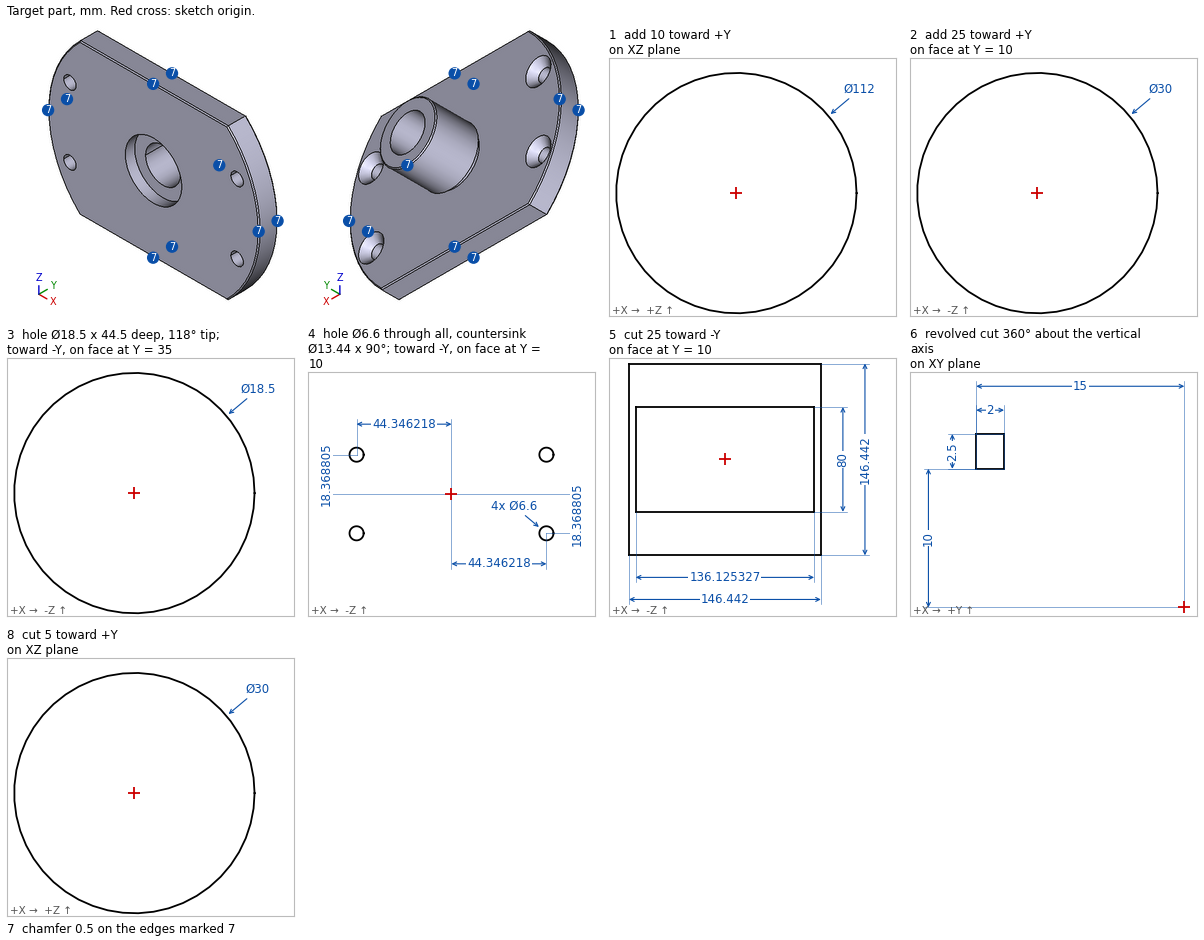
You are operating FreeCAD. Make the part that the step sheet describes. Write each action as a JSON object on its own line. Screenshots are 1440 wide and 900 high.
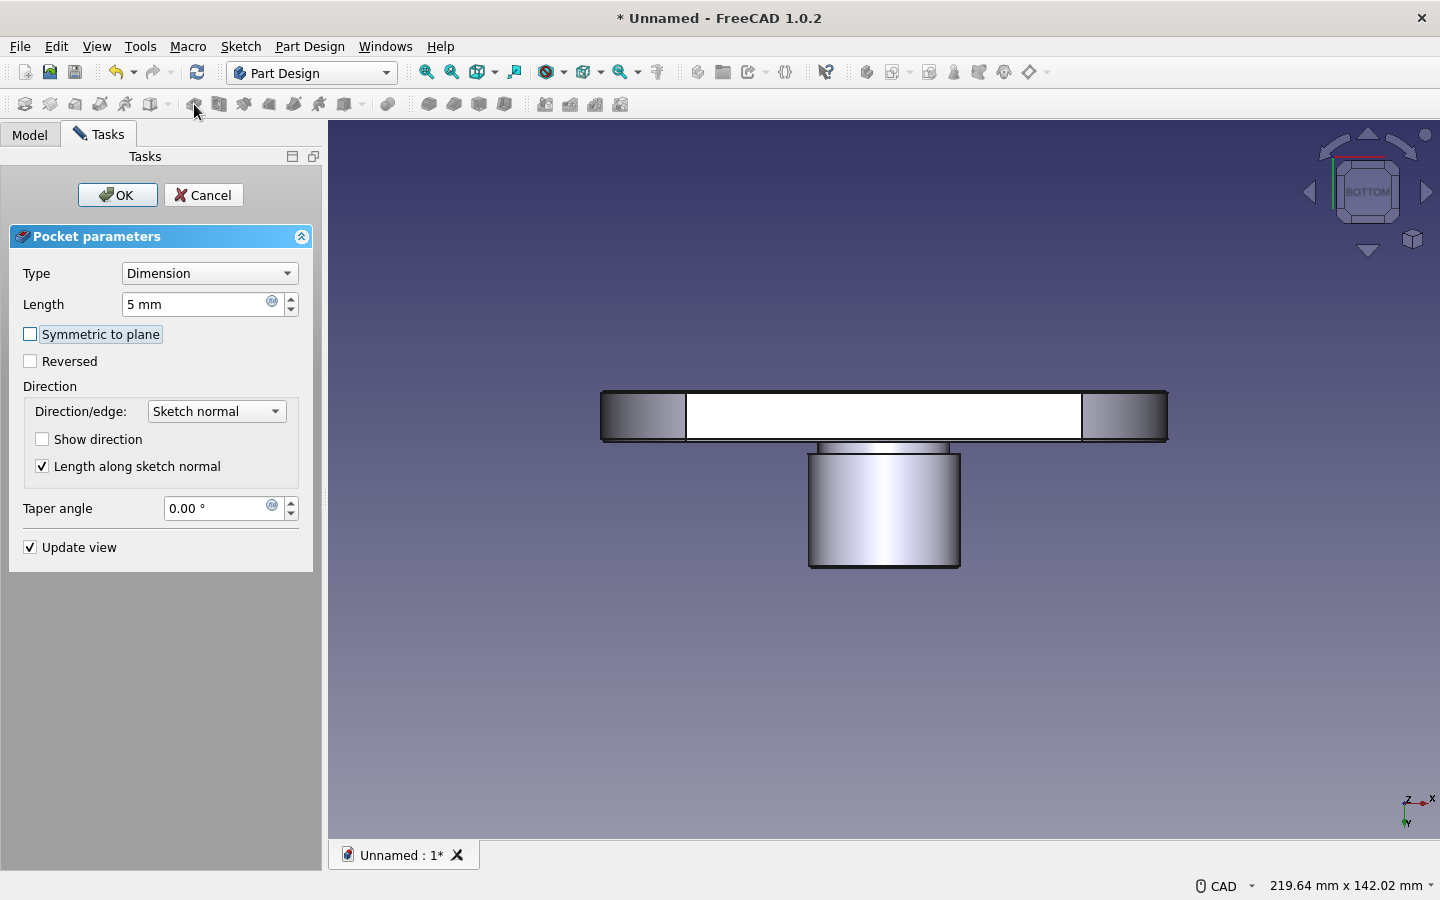
{"action": "left_click", "coordinate": [118, 195]}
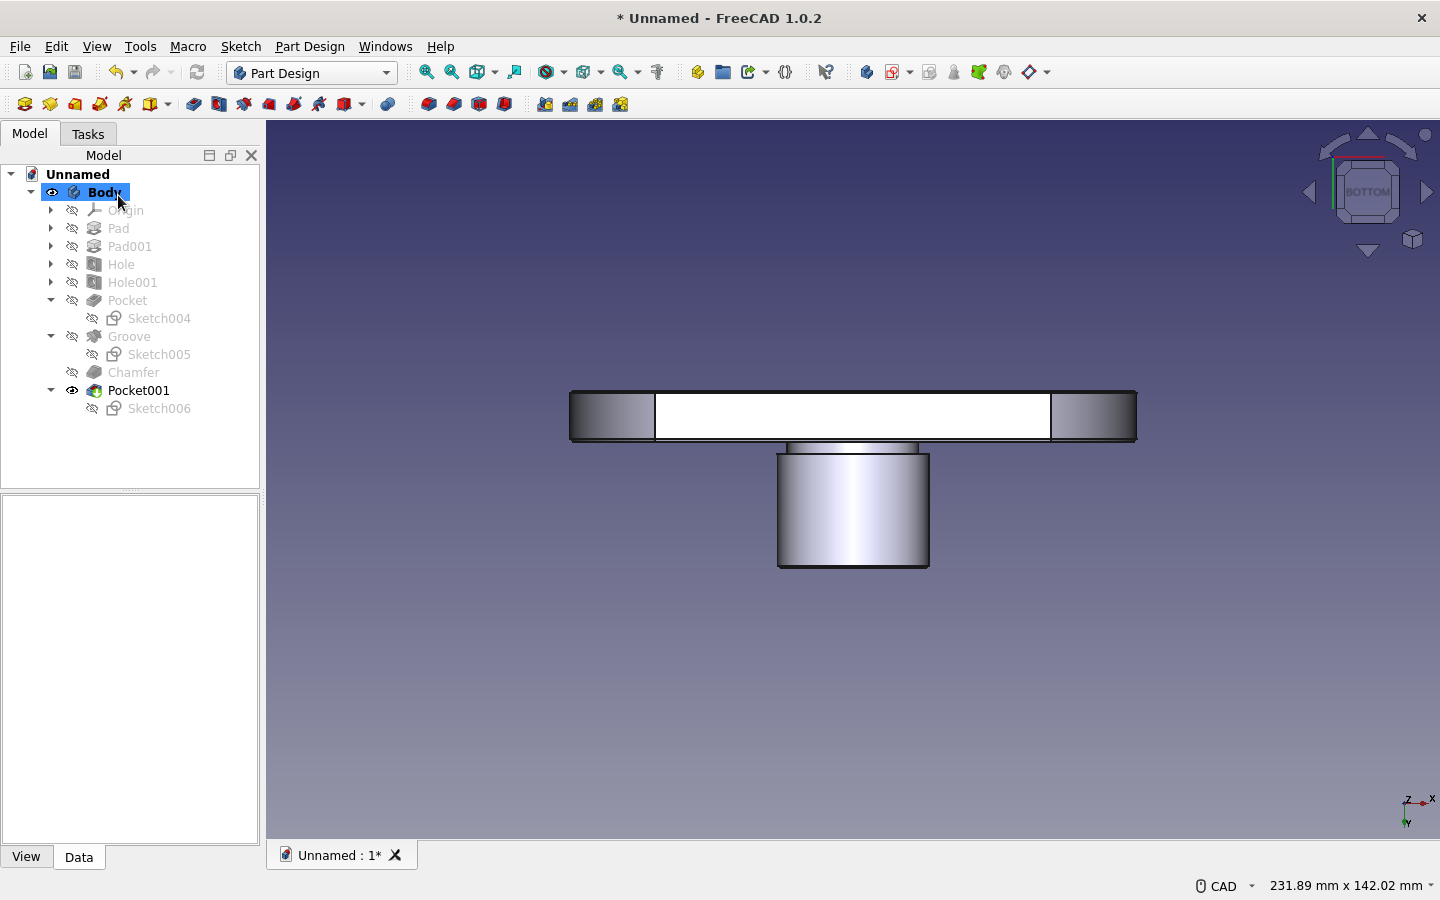
{"action": "key", "text": "0"}